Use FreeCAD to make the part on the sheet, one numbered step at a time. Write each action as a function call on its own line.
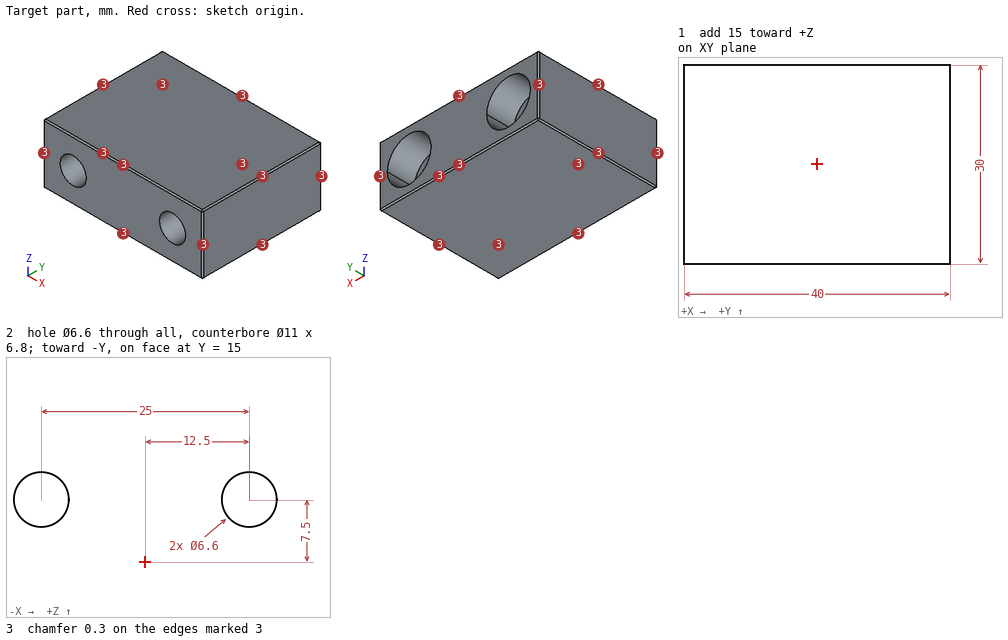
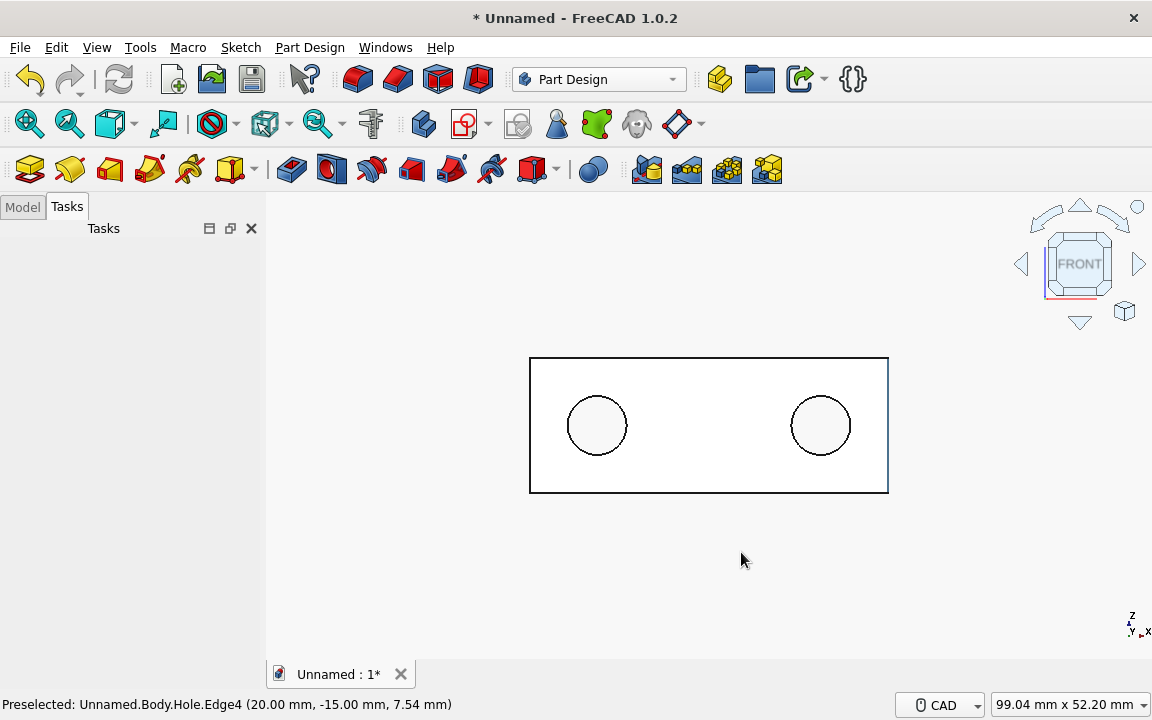
click(30, 124)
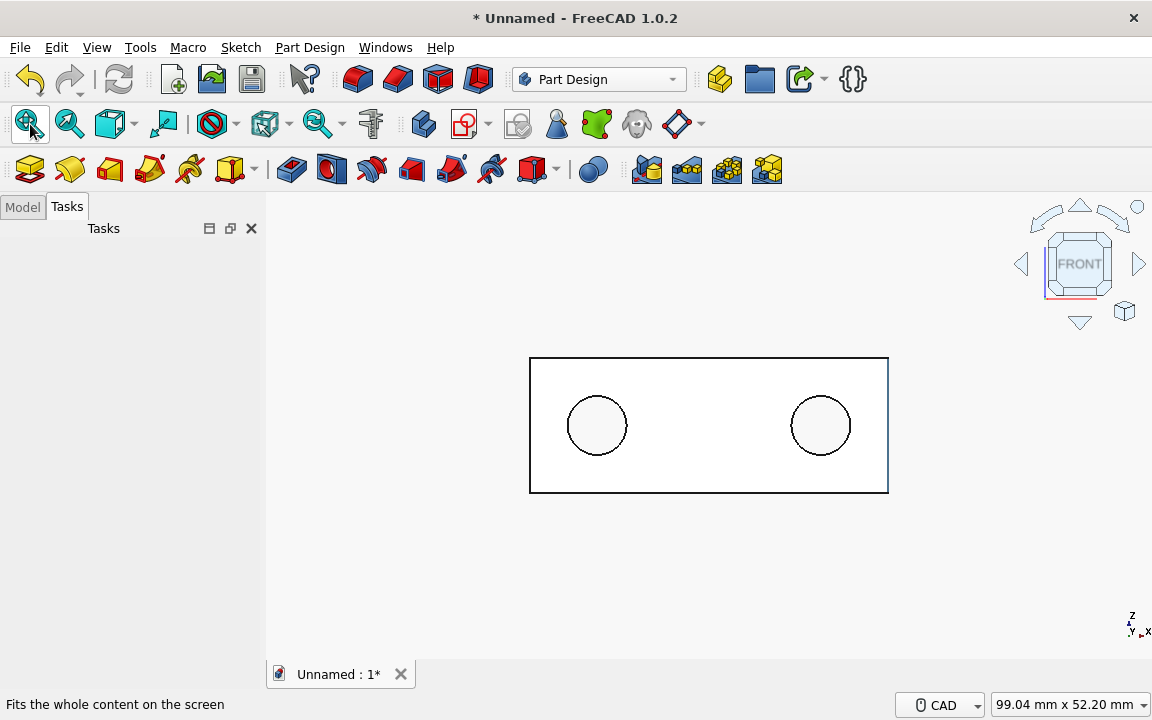
click(530, 425, ctrl)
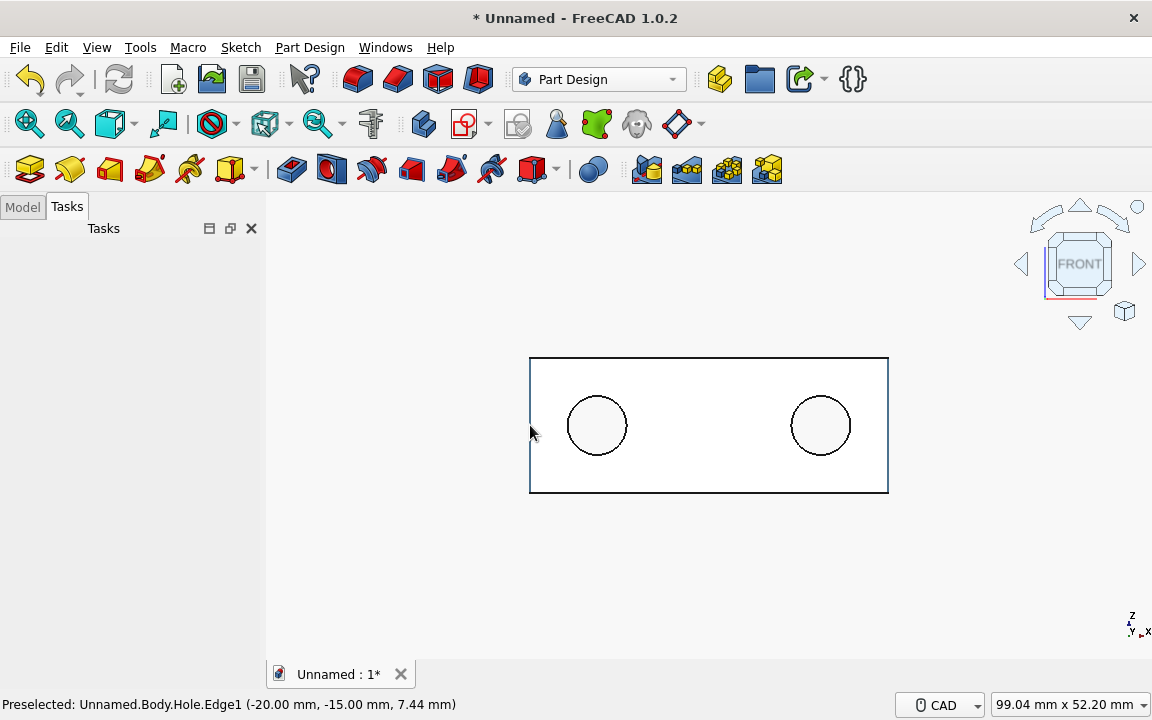
key(3)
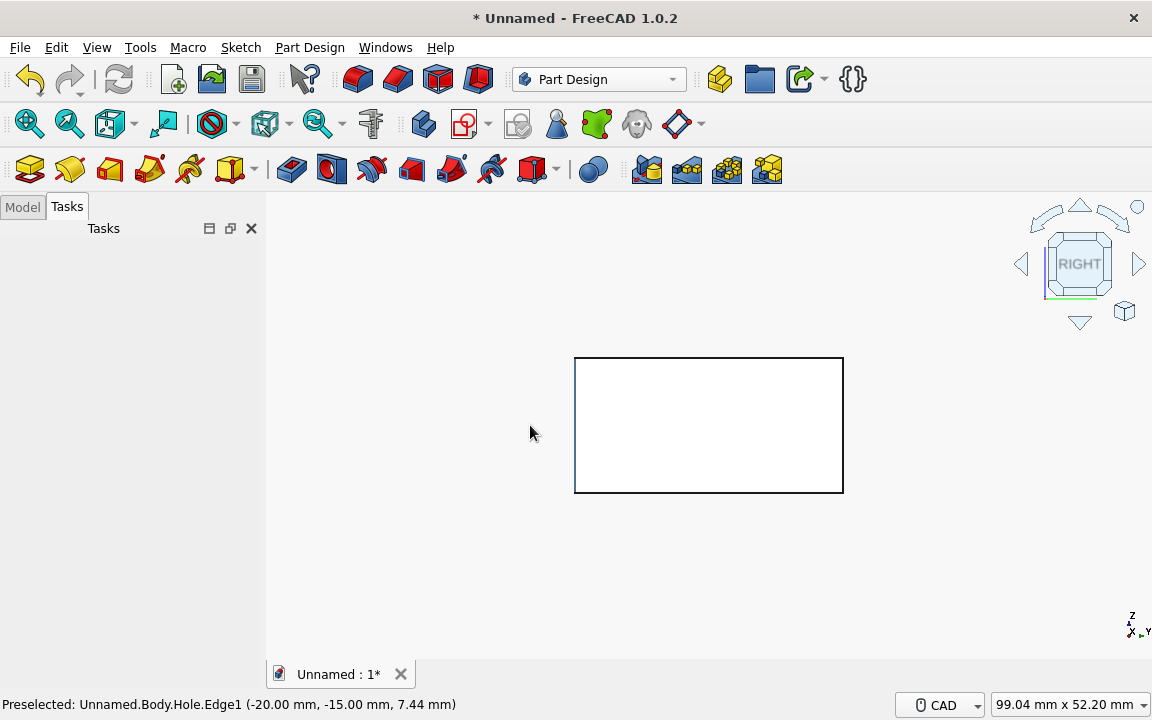
click(30, 124)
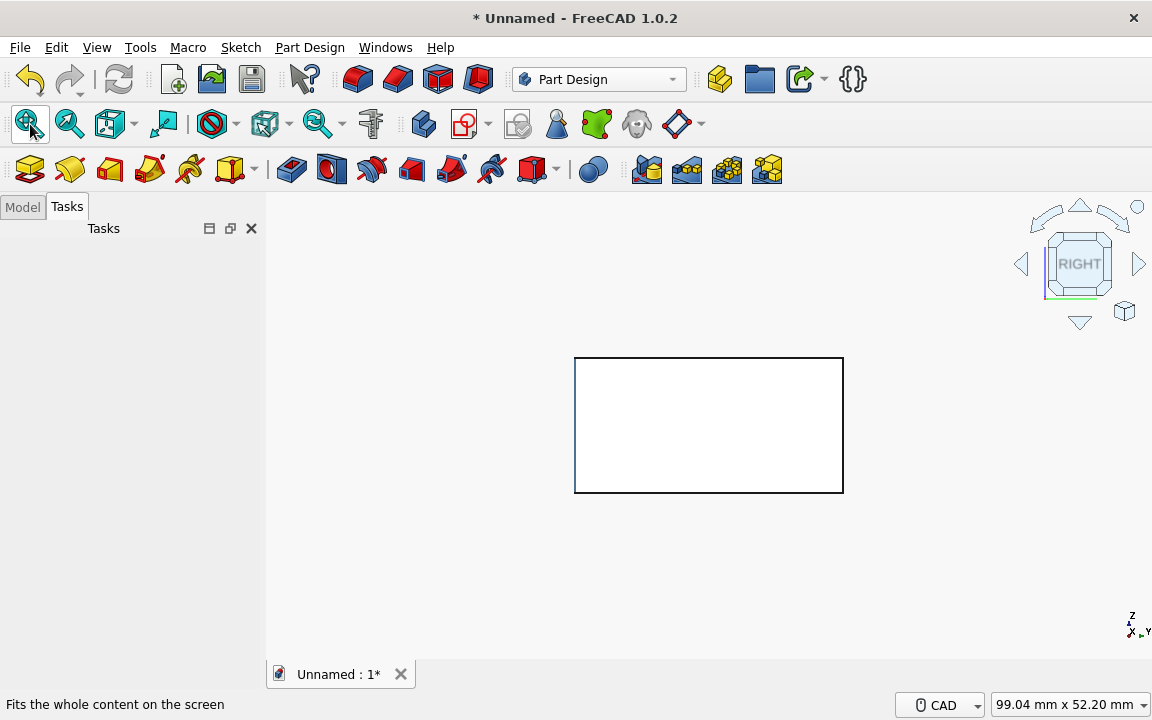
click(843, 424, ctrl)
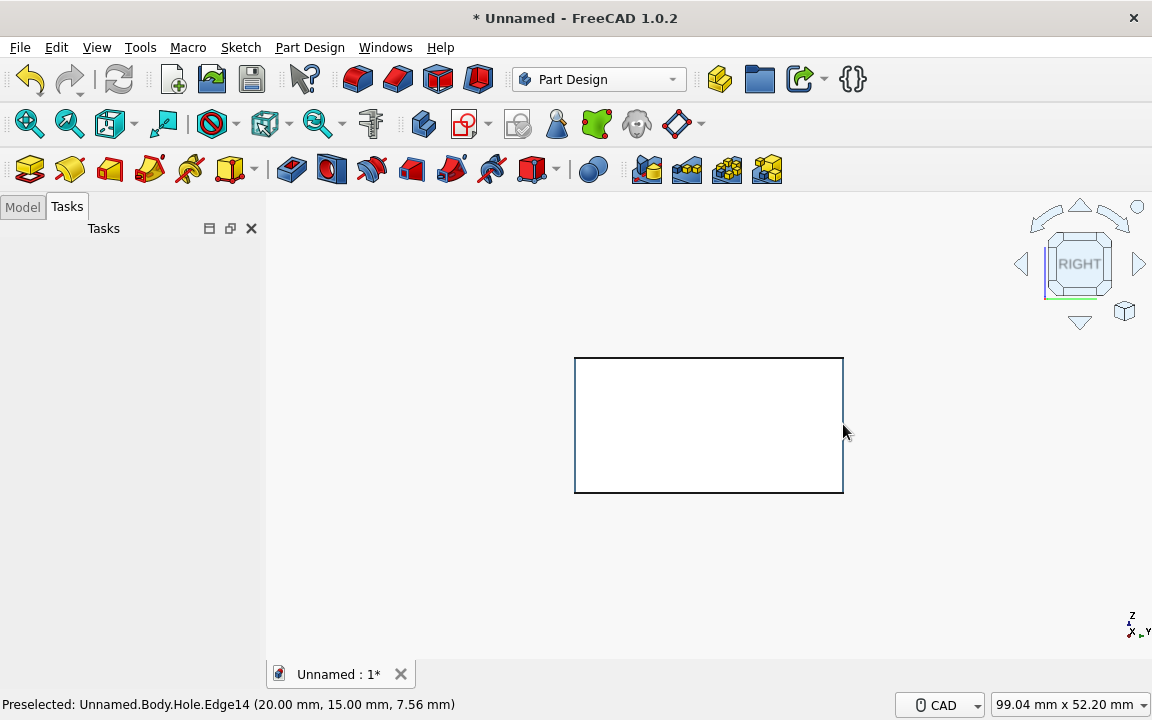
key(5)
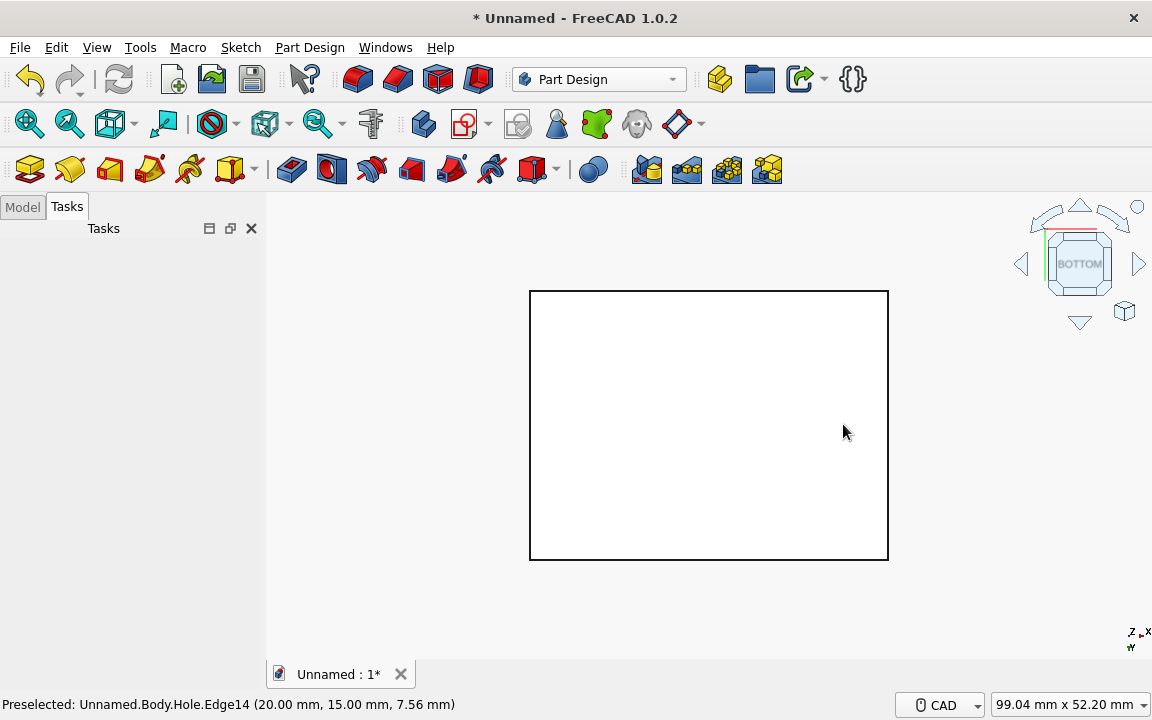
click(709, 424, ctrl)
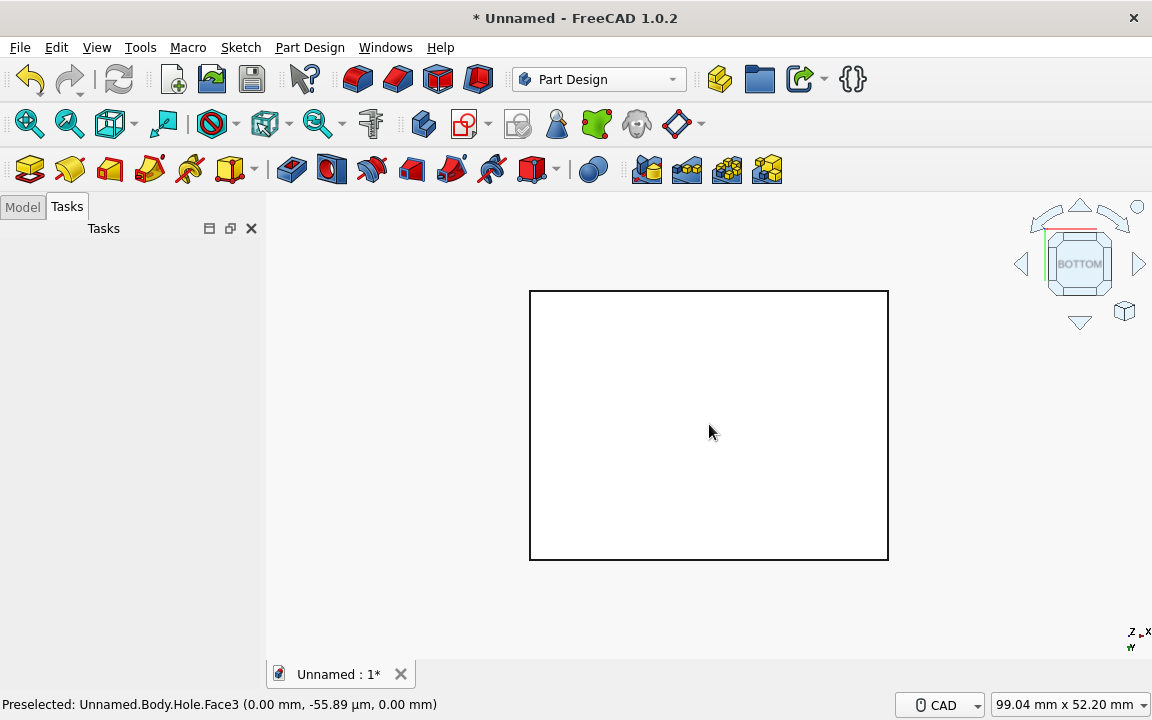
click(398, 80)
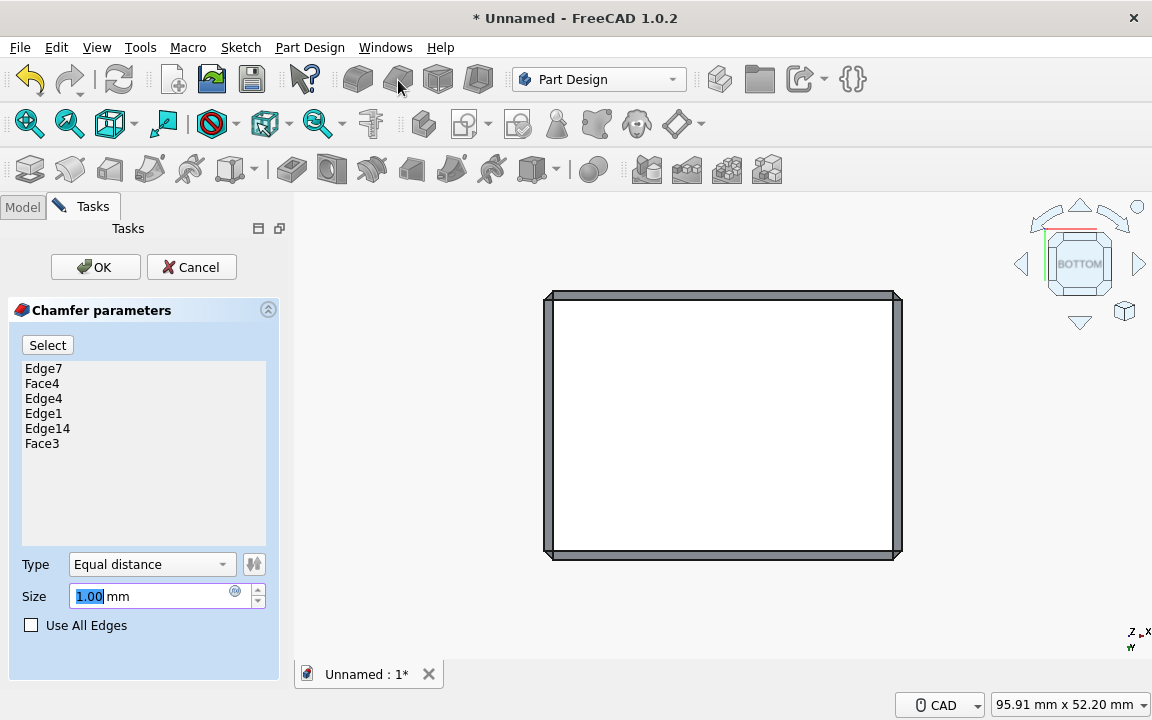
text(0.3)
key(Tab)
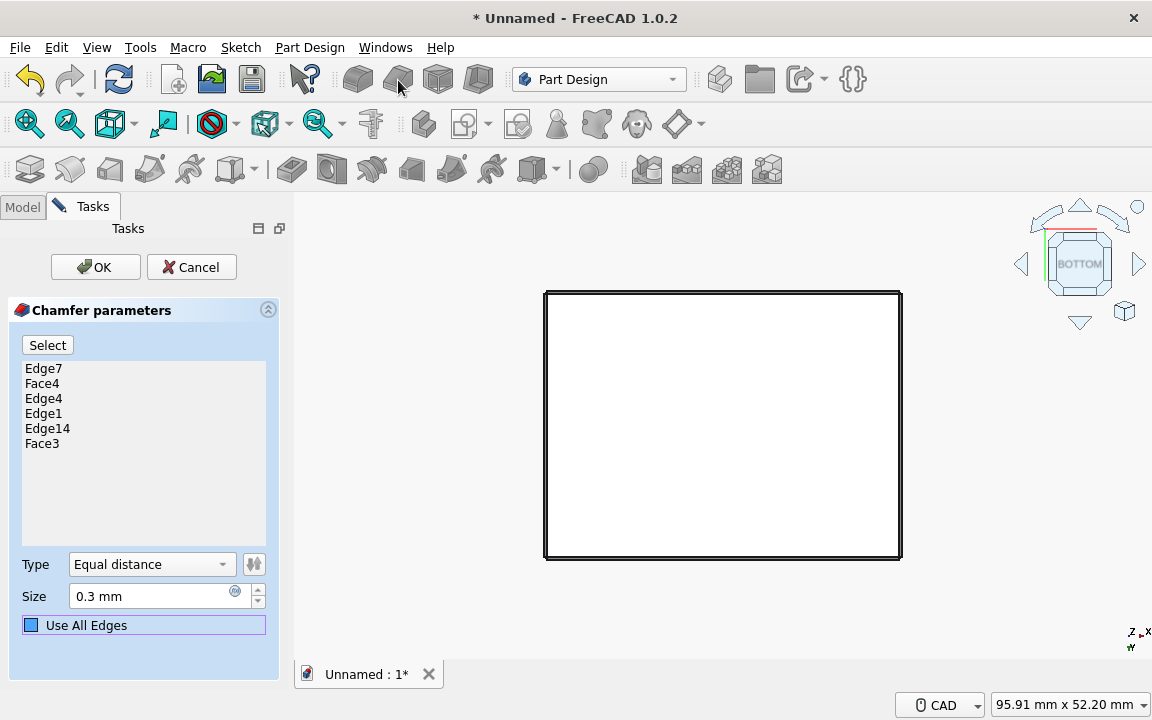
click(96, 267)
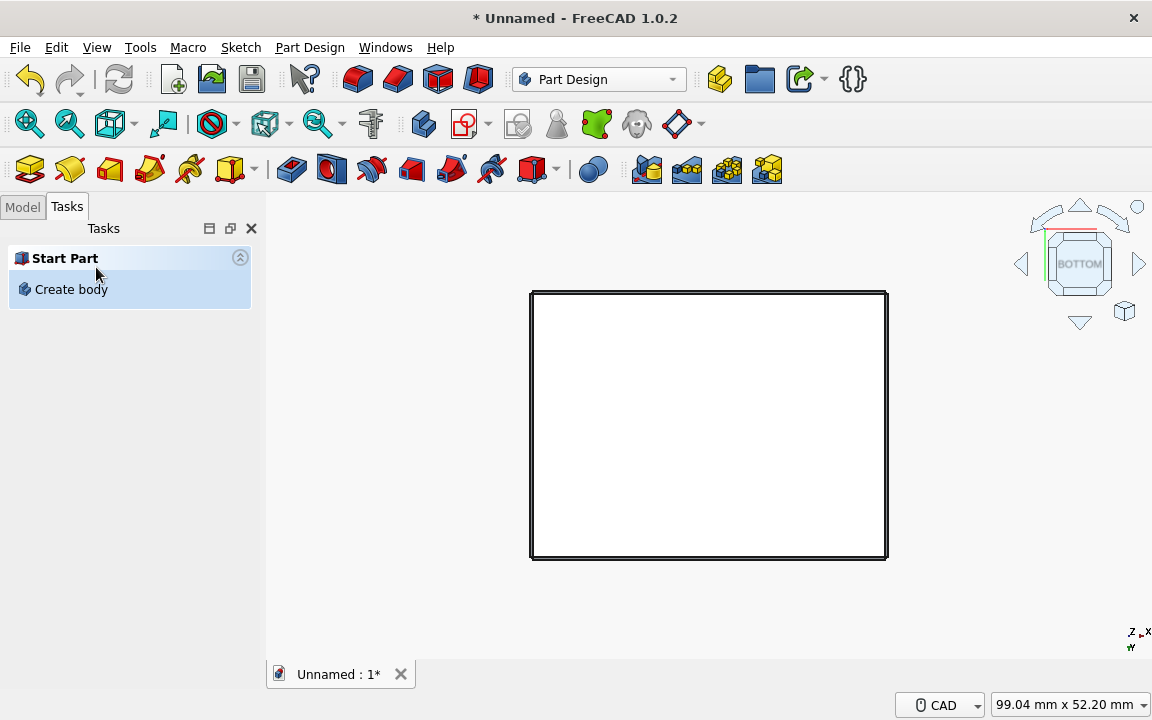
key(0)